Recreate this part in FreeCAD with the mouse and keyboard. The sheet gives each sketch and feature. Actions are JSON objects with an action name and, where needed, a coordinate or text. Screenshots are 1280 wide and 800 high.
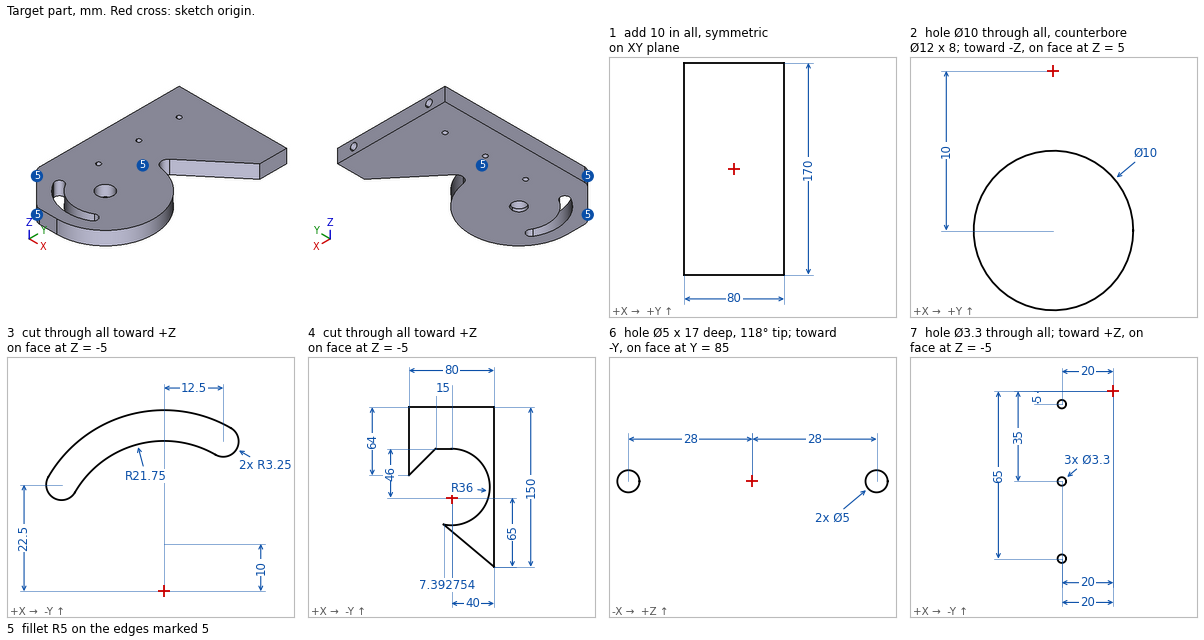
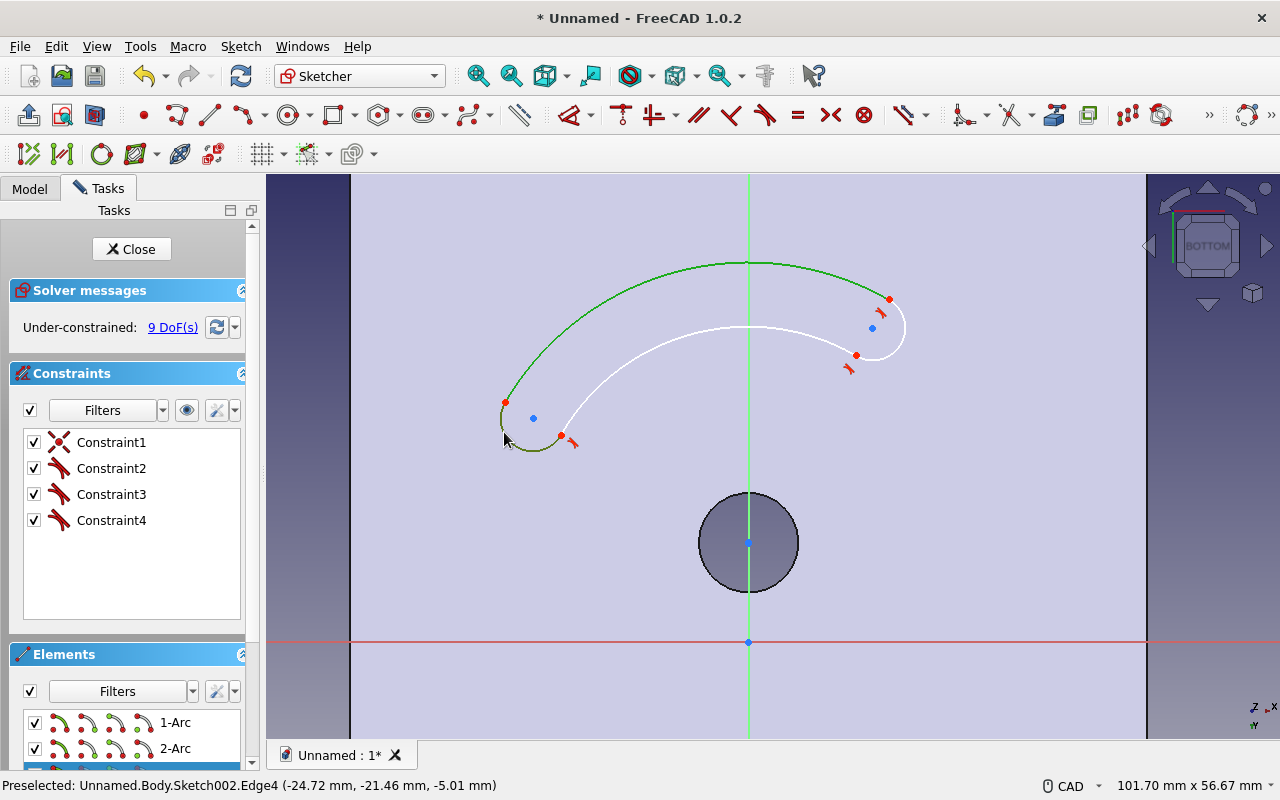
{"action": "key", "text": "t"}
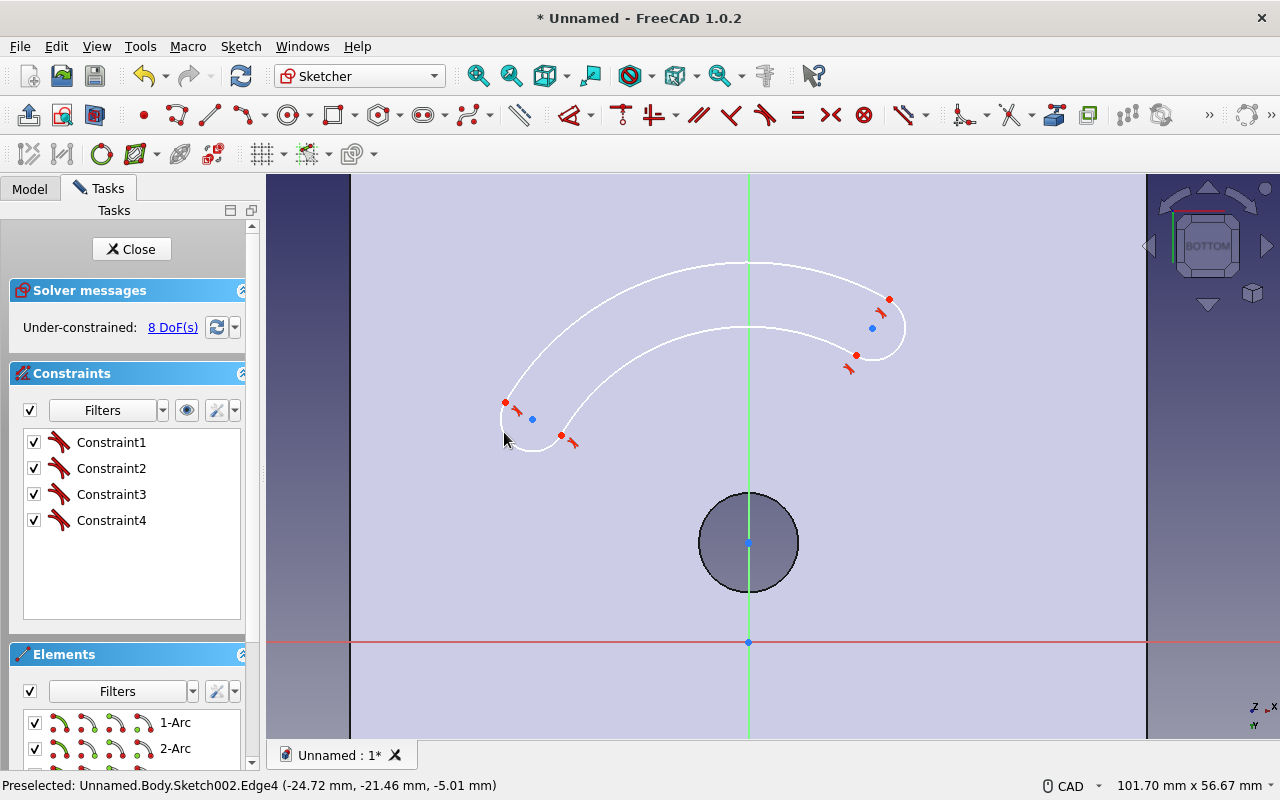
{"action": "scroll", "coordinate": [760, 327], "scroll_direction": "up", "scroll_amount": 2}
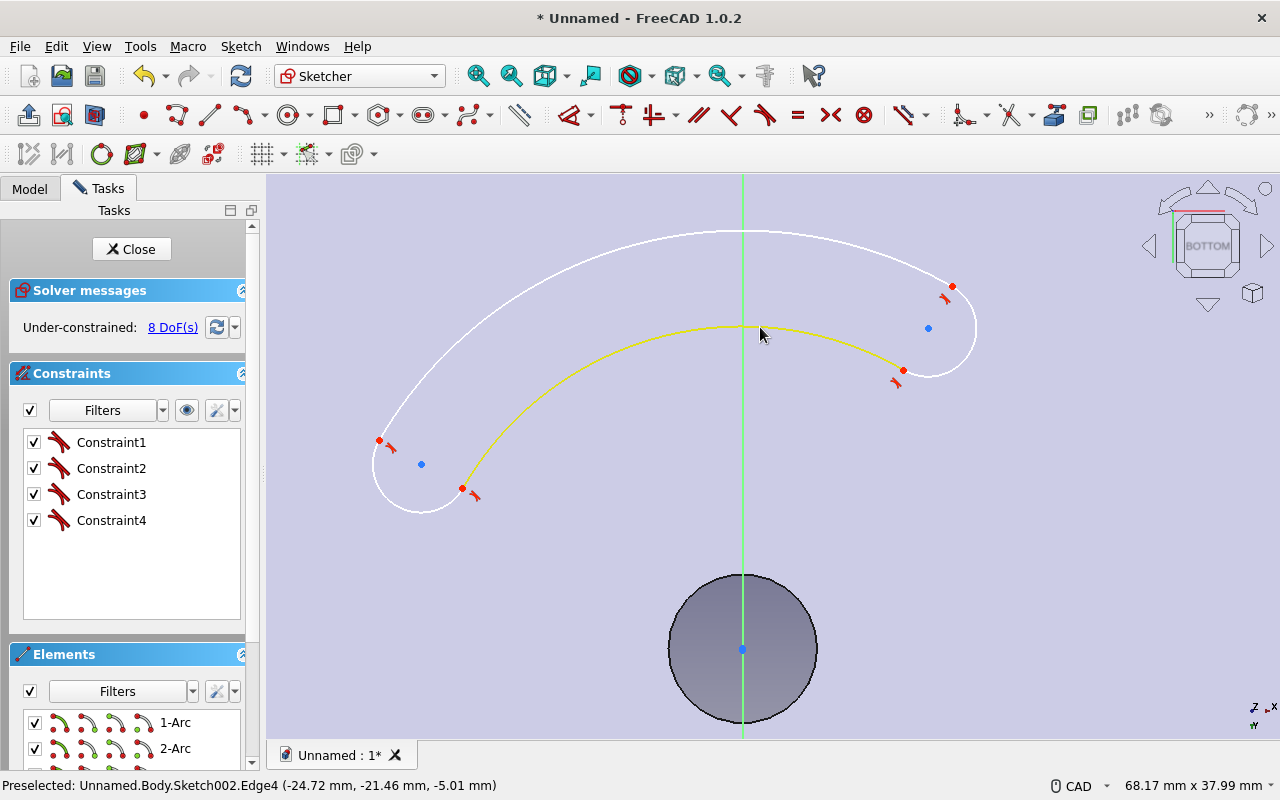
{"action": "left_click", "coordinate": [759, 327]}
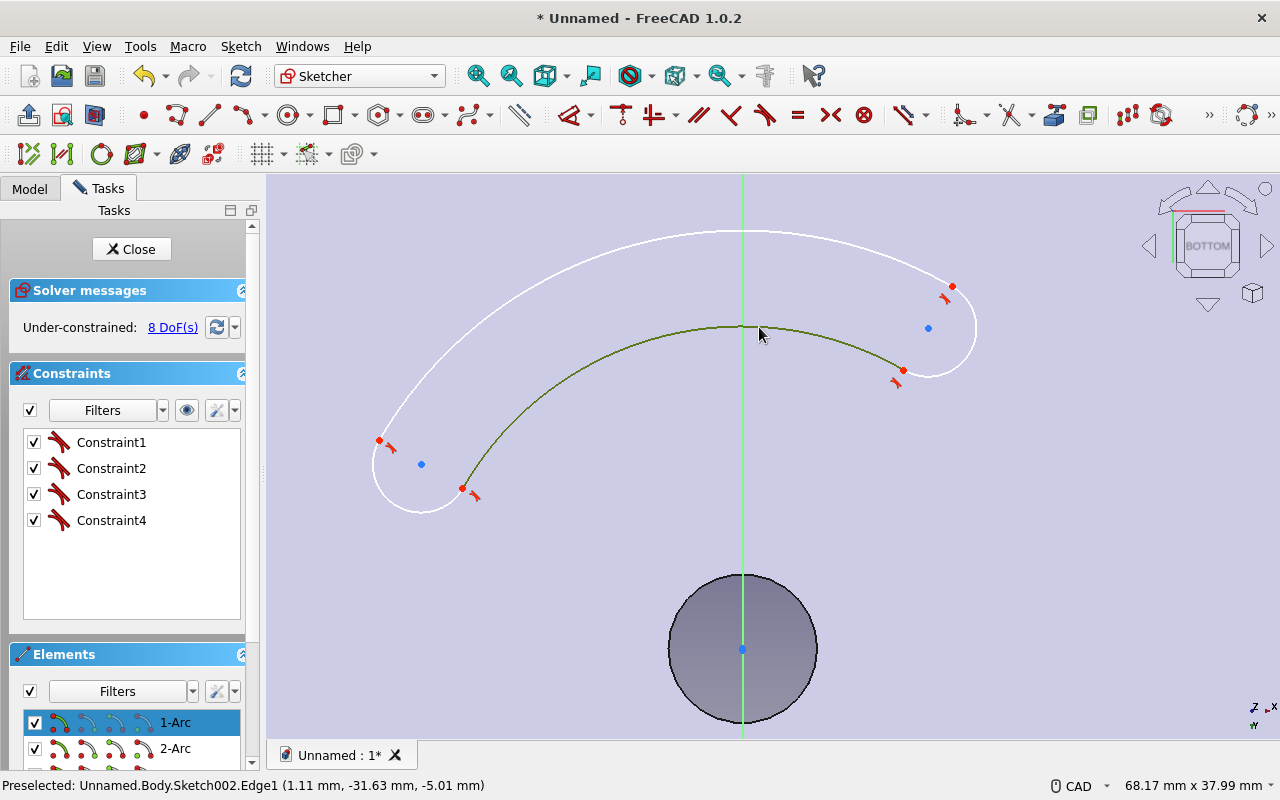
{"action": "left_click", "coordinate": [764, 231]}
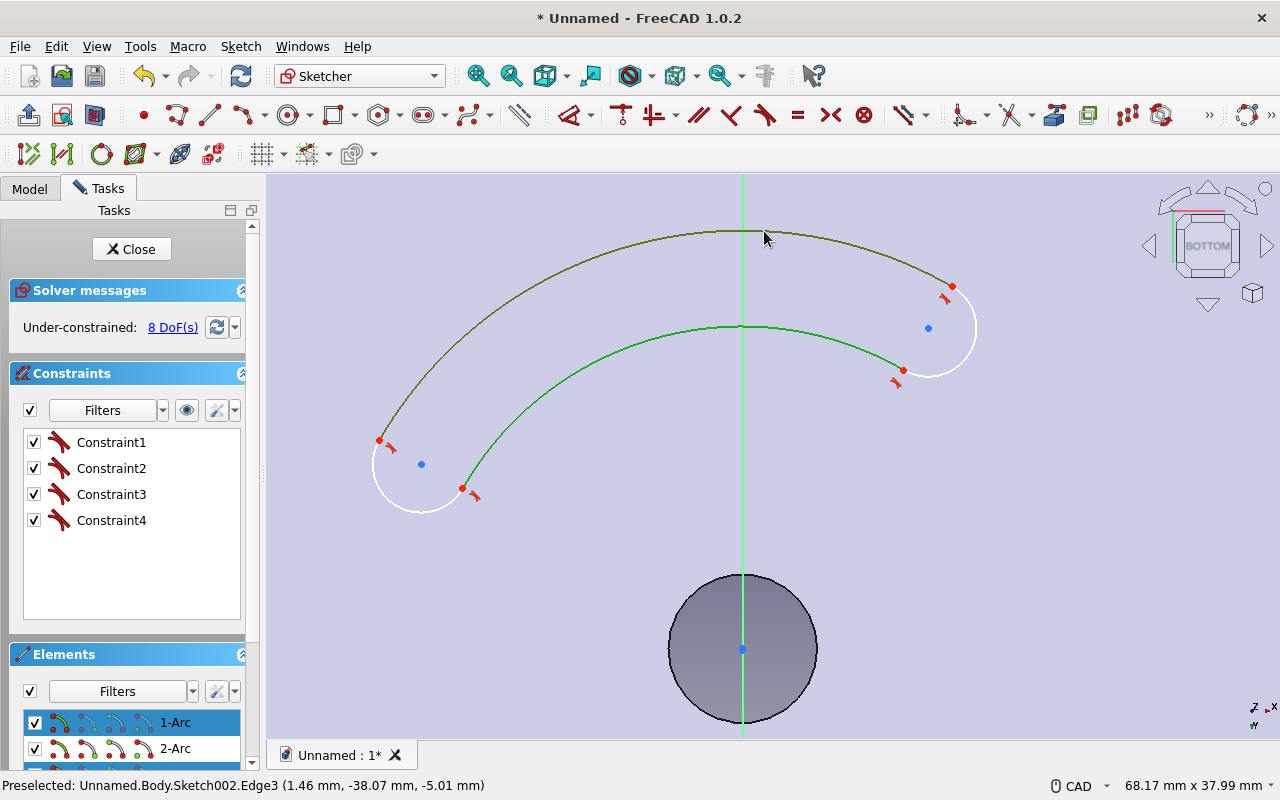
{"action": "left_click", "coordinate": [621, 116]}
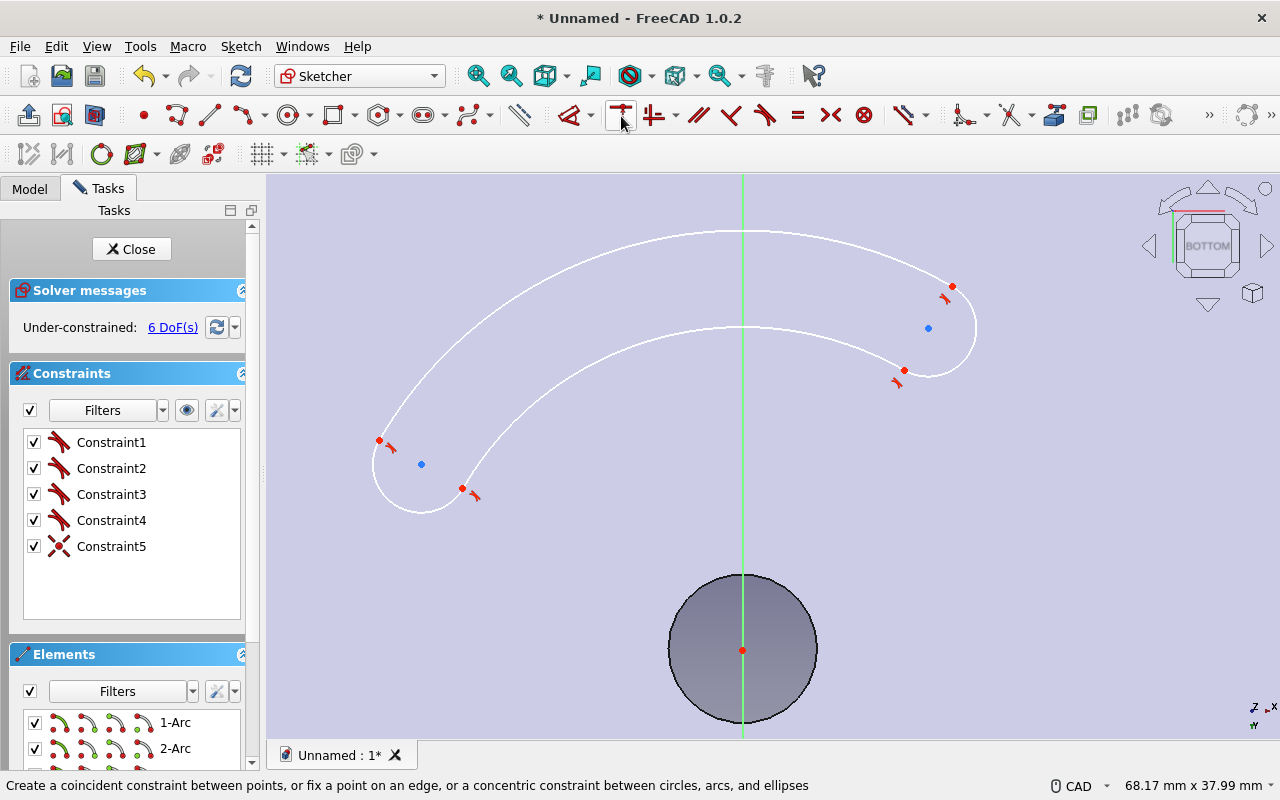
{"action": "left_click", "coordinate": [743, 650]}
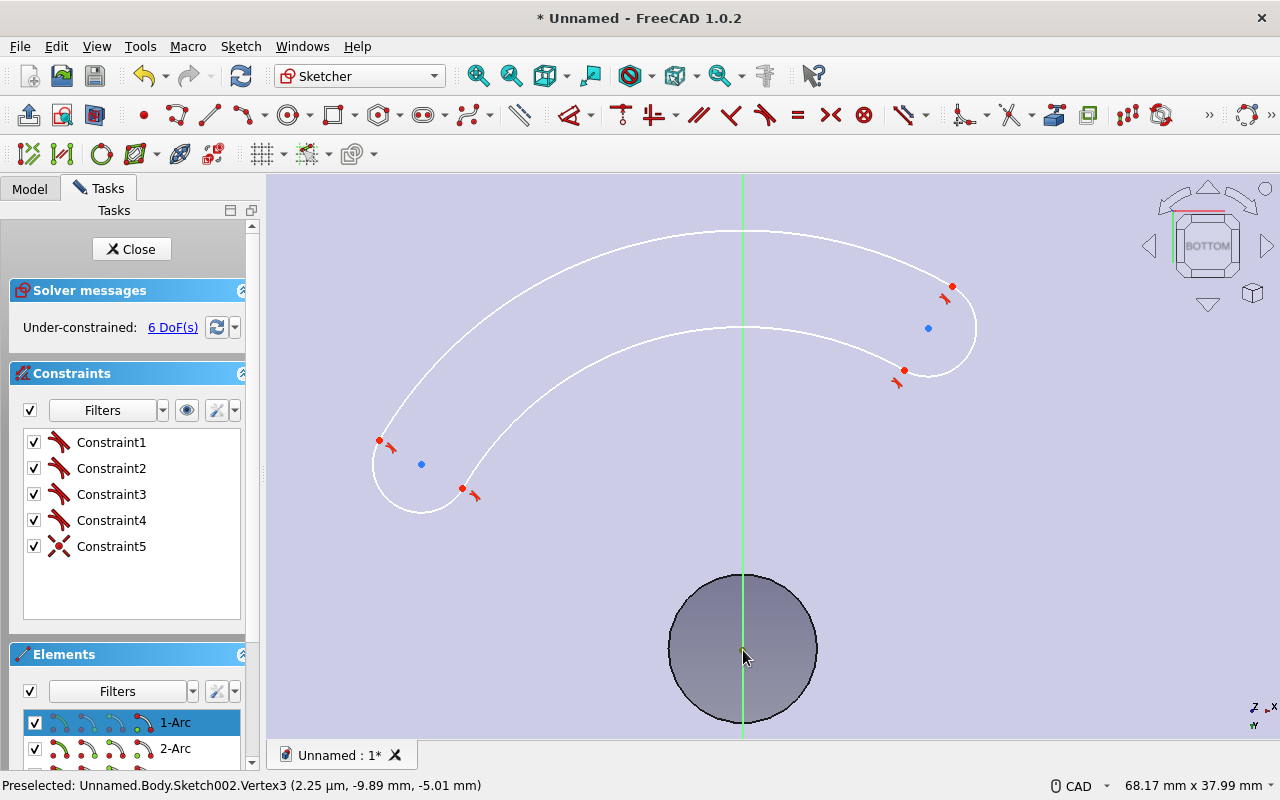
{"action": "left_click", "coordinate": [743, 675]}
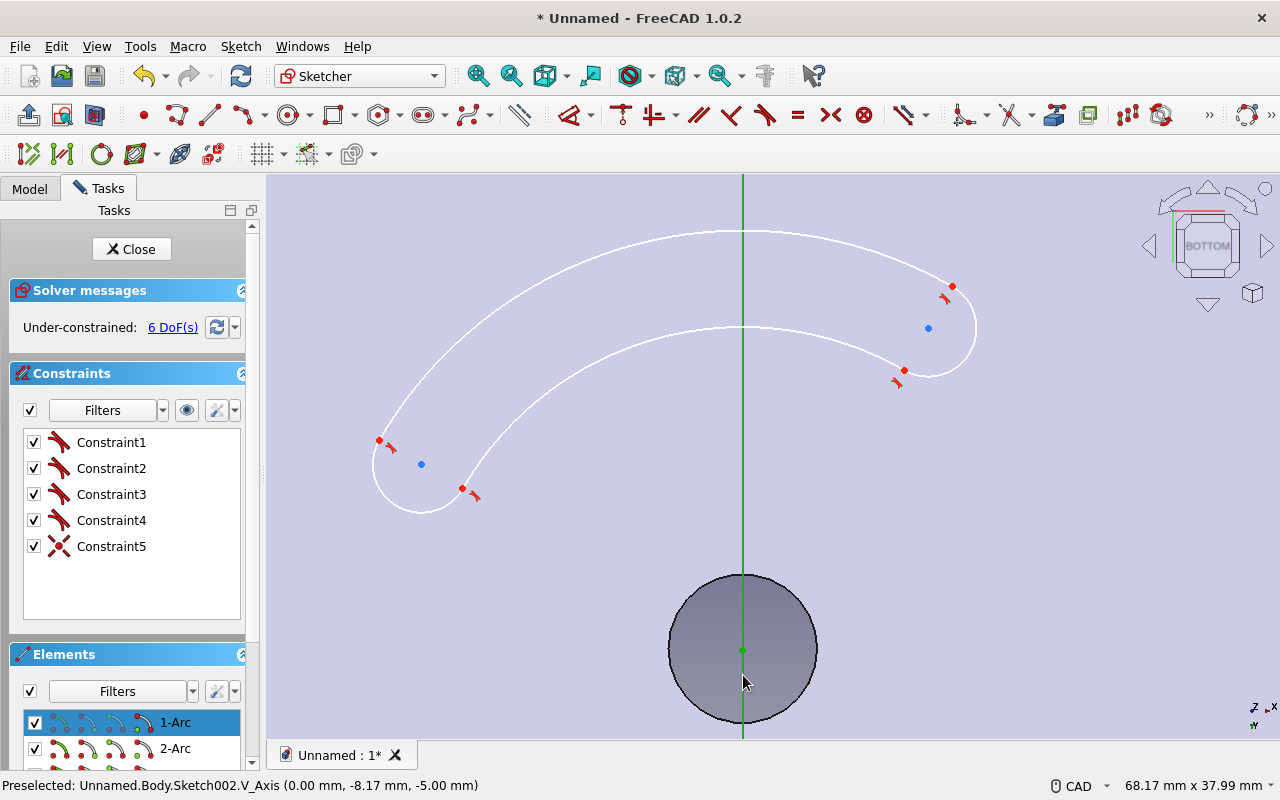
{"action": "left_click", "coordinate": [621, 116]}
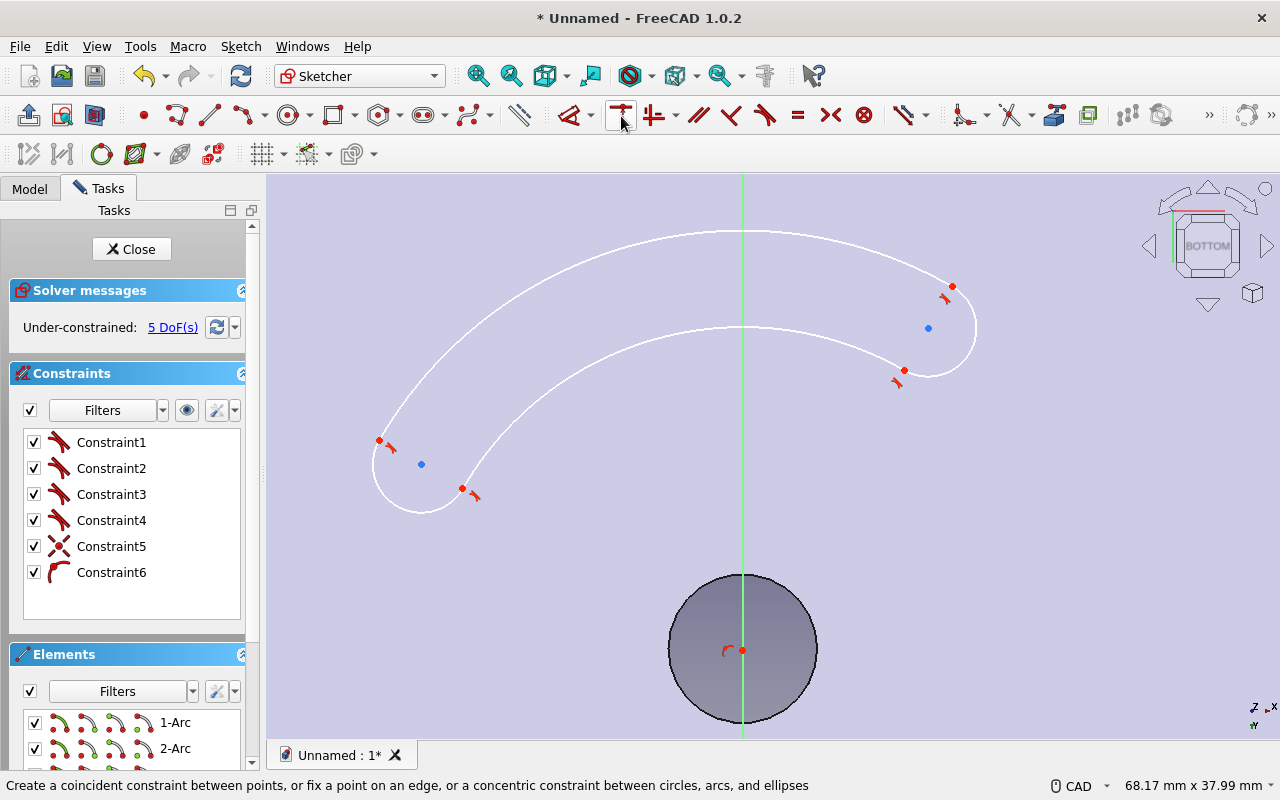
{"action": "key", "text": "d"}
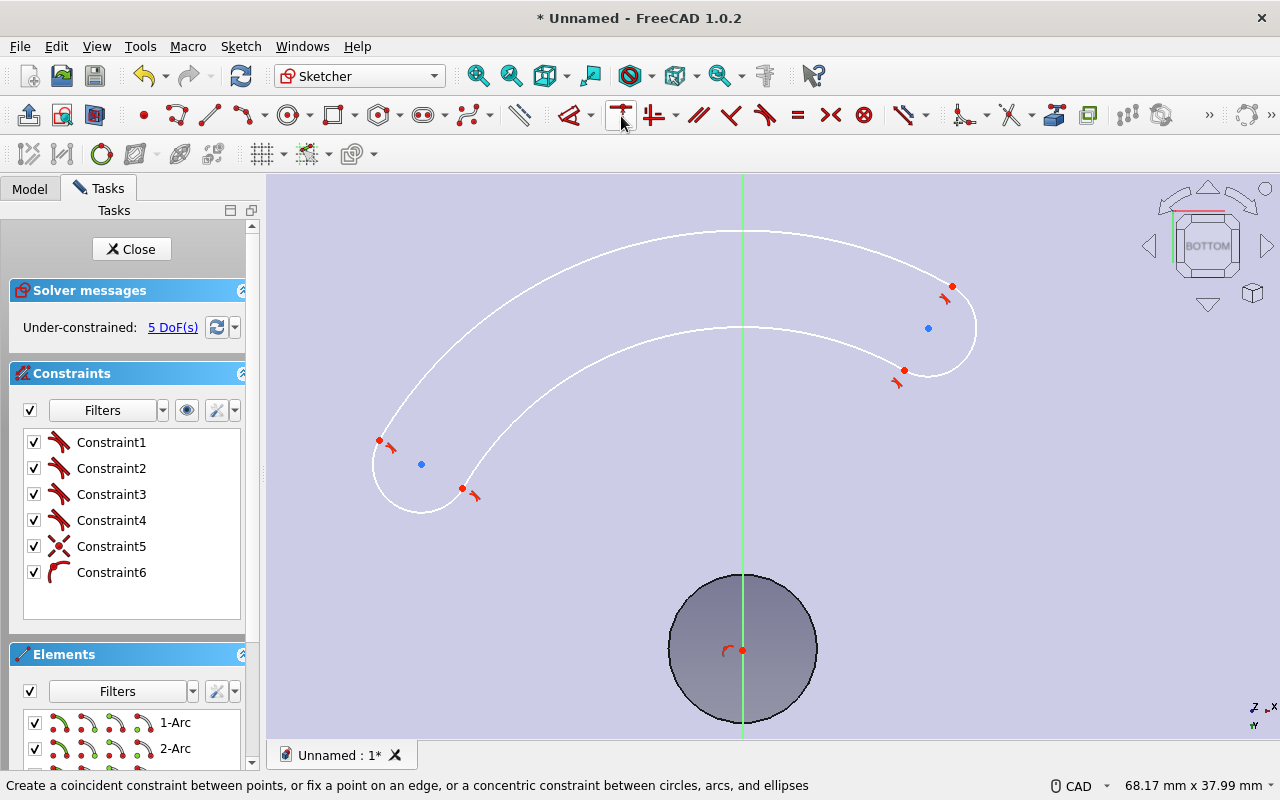
{"action": "left_click", "coordinate": [759, 328]}
{"action": "left_click", "coordinate": [761, 296]}